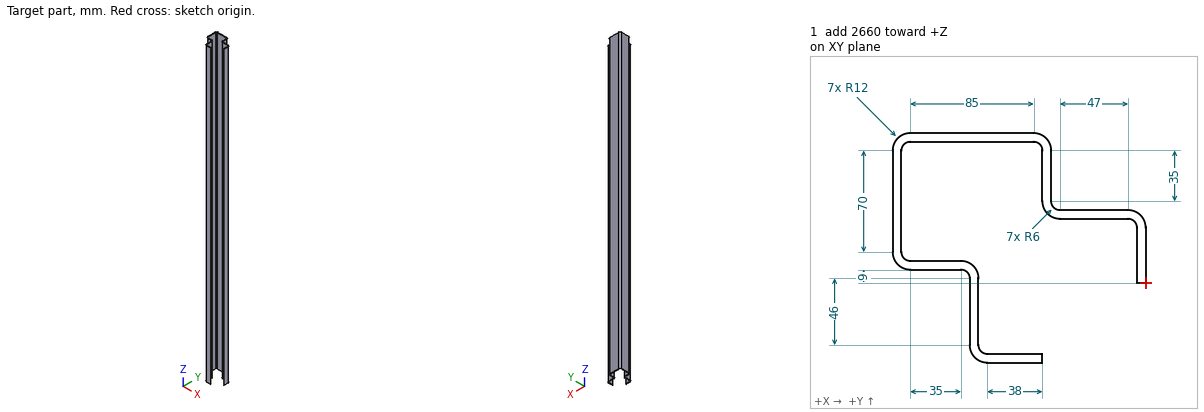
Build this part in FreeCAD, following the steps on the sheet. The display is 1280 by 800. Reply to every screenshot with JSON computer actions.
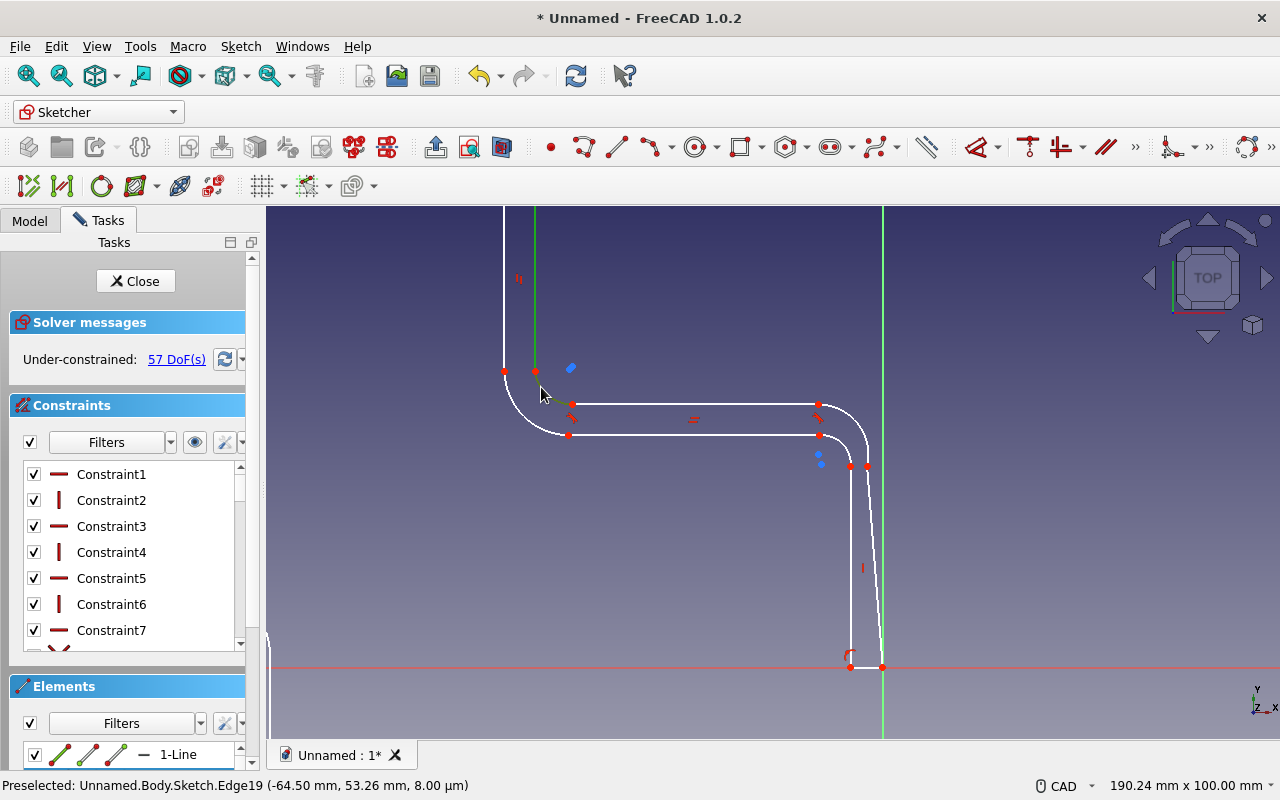
{"action": "key", "text": "t"}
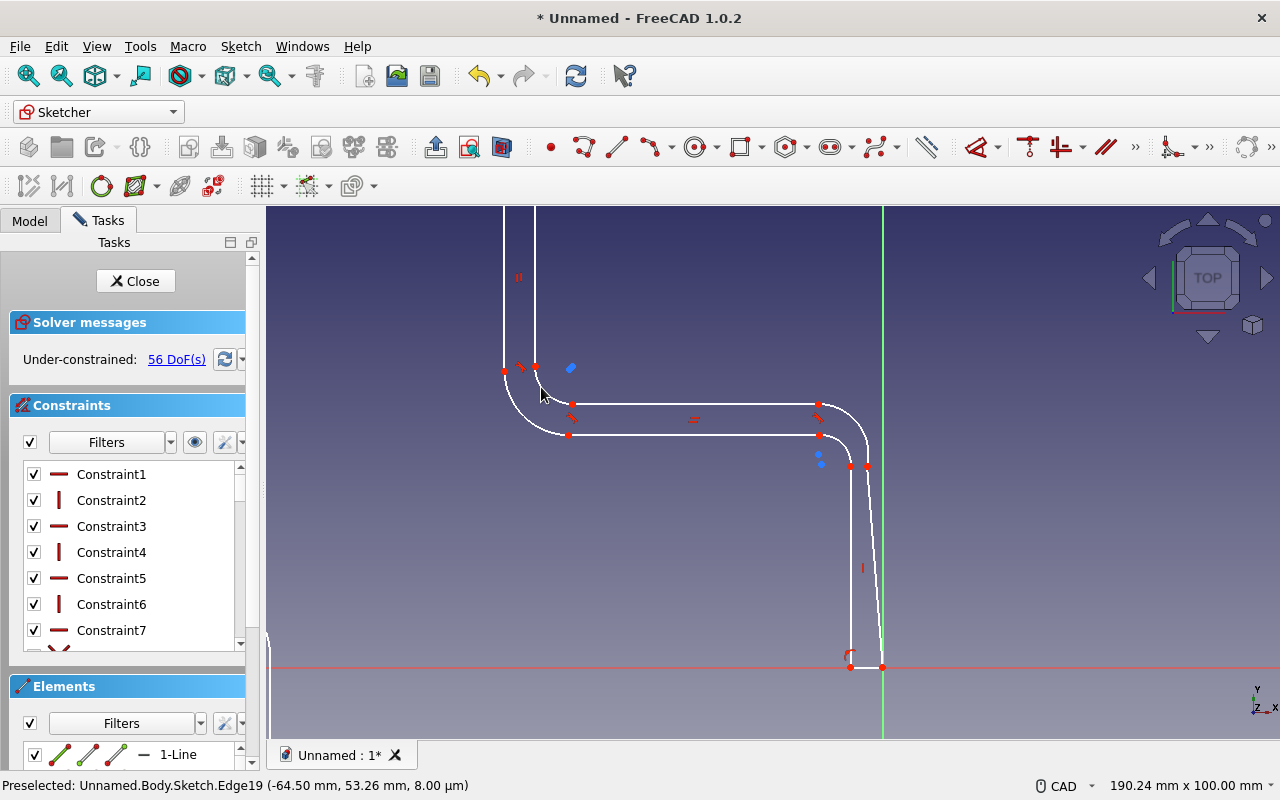
{"action": "left_click", "coordinate": [535, 313]}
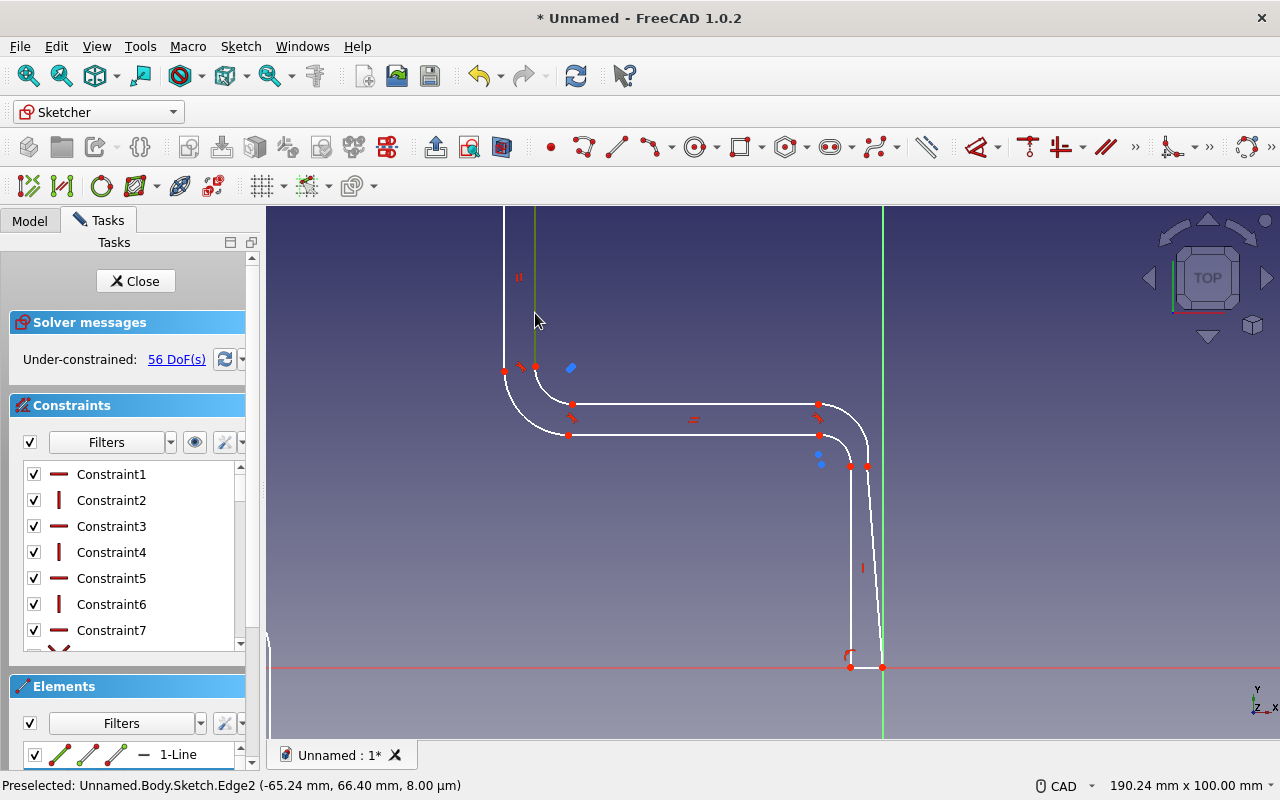
{"action": "scroll", "coordinate": [871, 433], "scroll_direction": "down", "scroll_amount": 5}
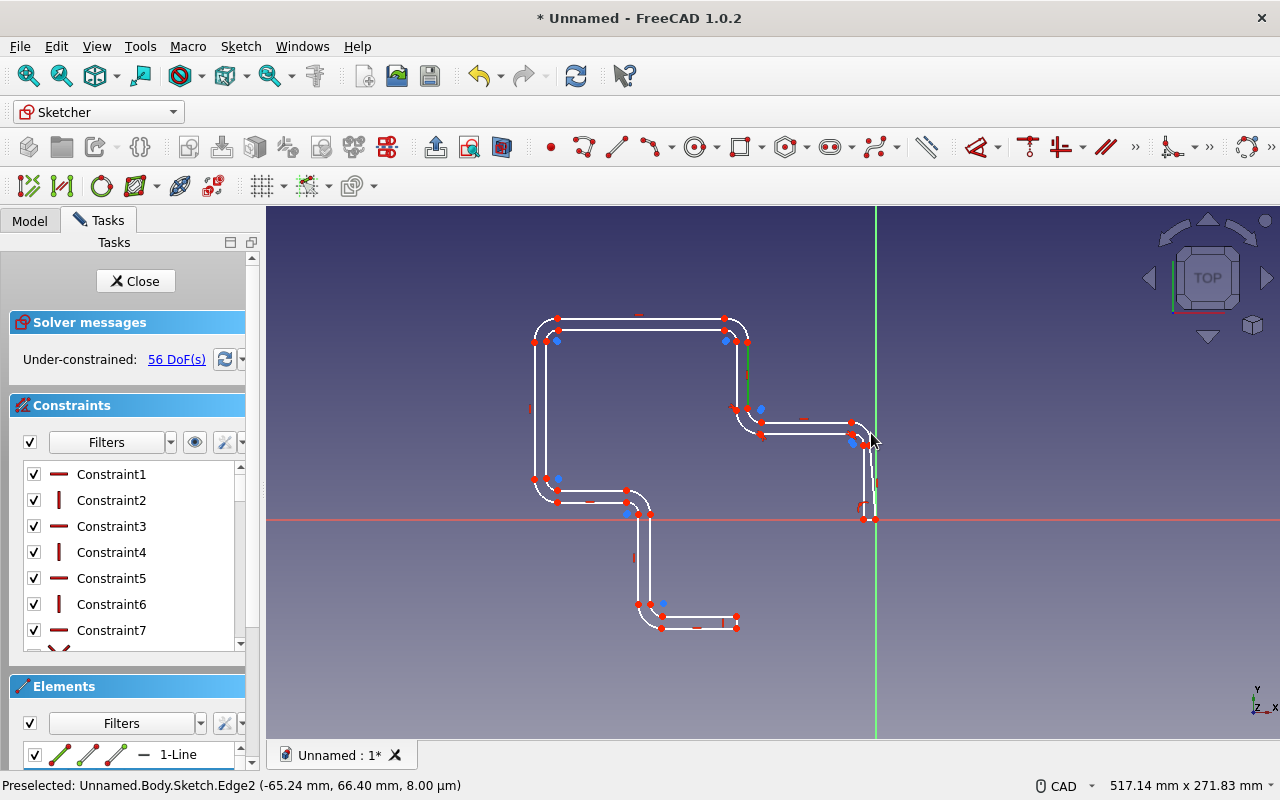
{"action": "scroll", "coordinate": [746, 332], "scroll_direction": "up", "scroll_amount": 2}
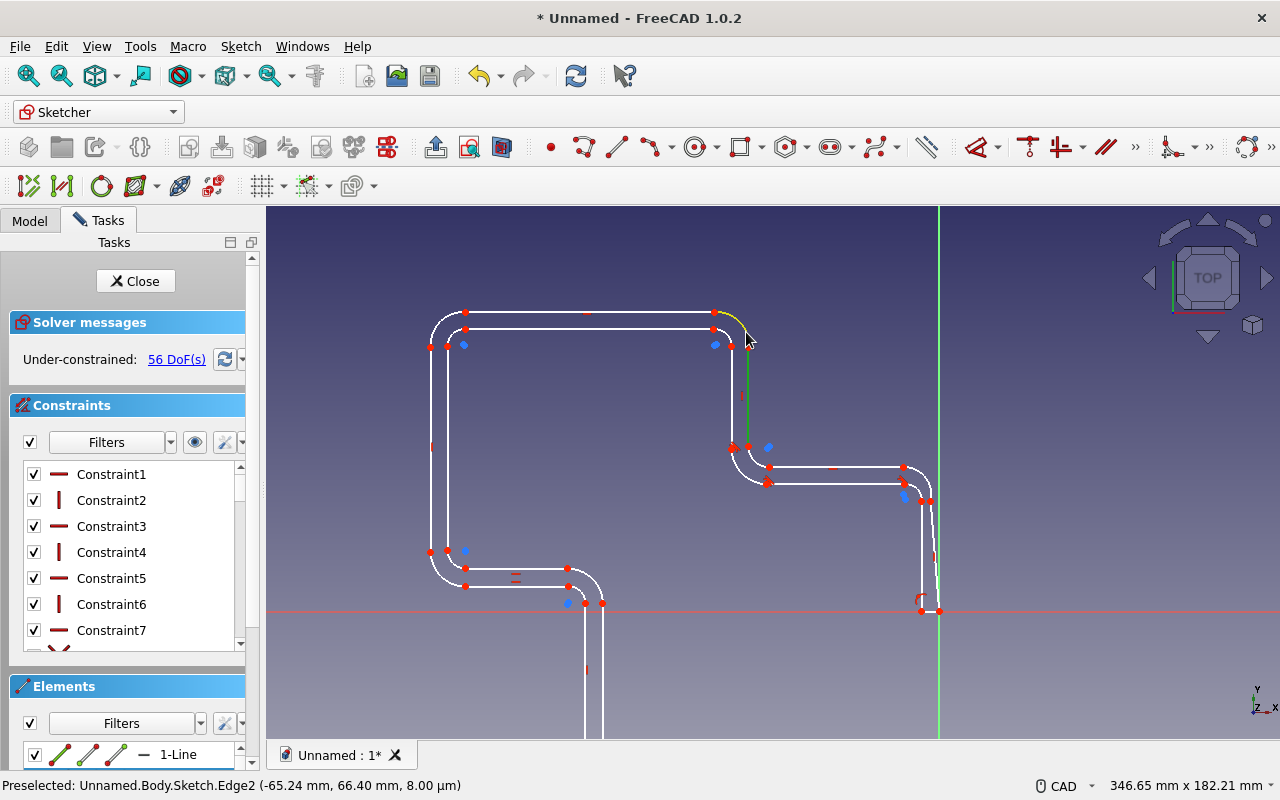
{"action": "left_click", "coordinate": [746, 331]}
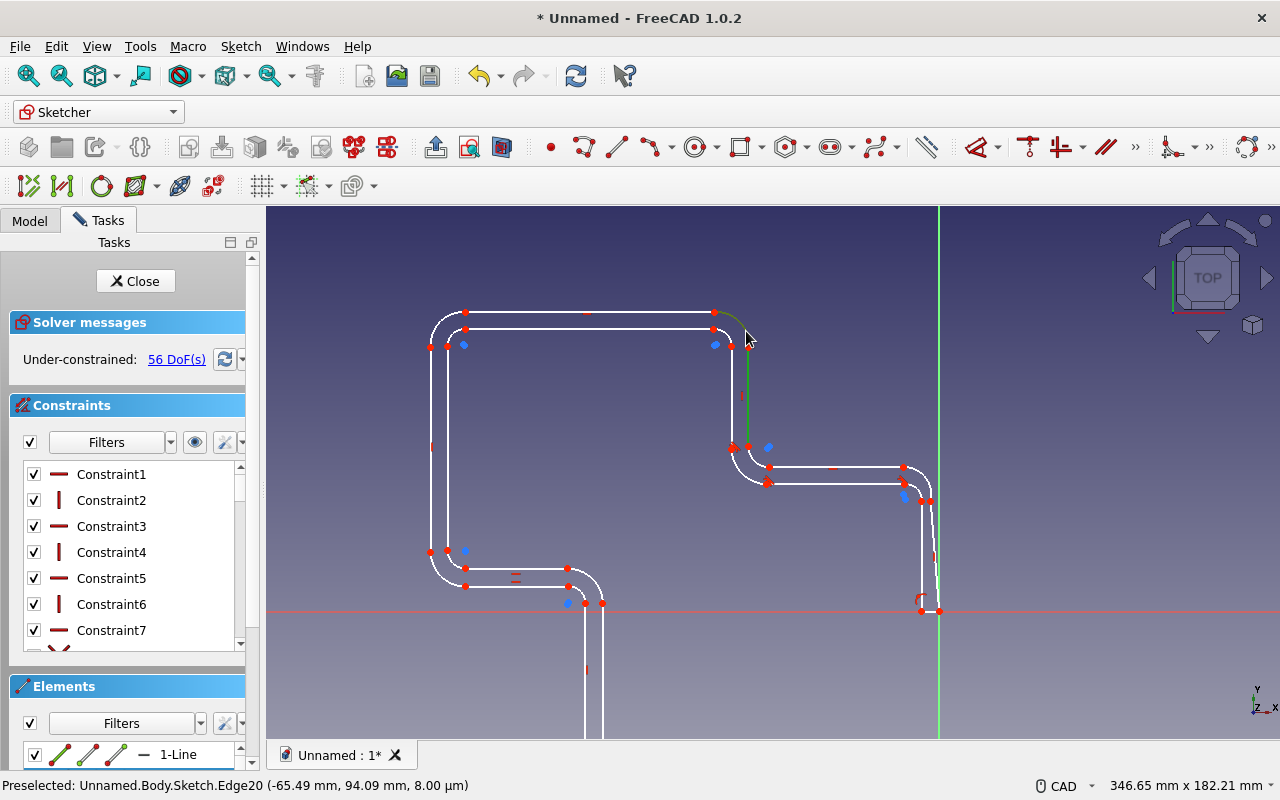
{"action": "key", "text": "t"}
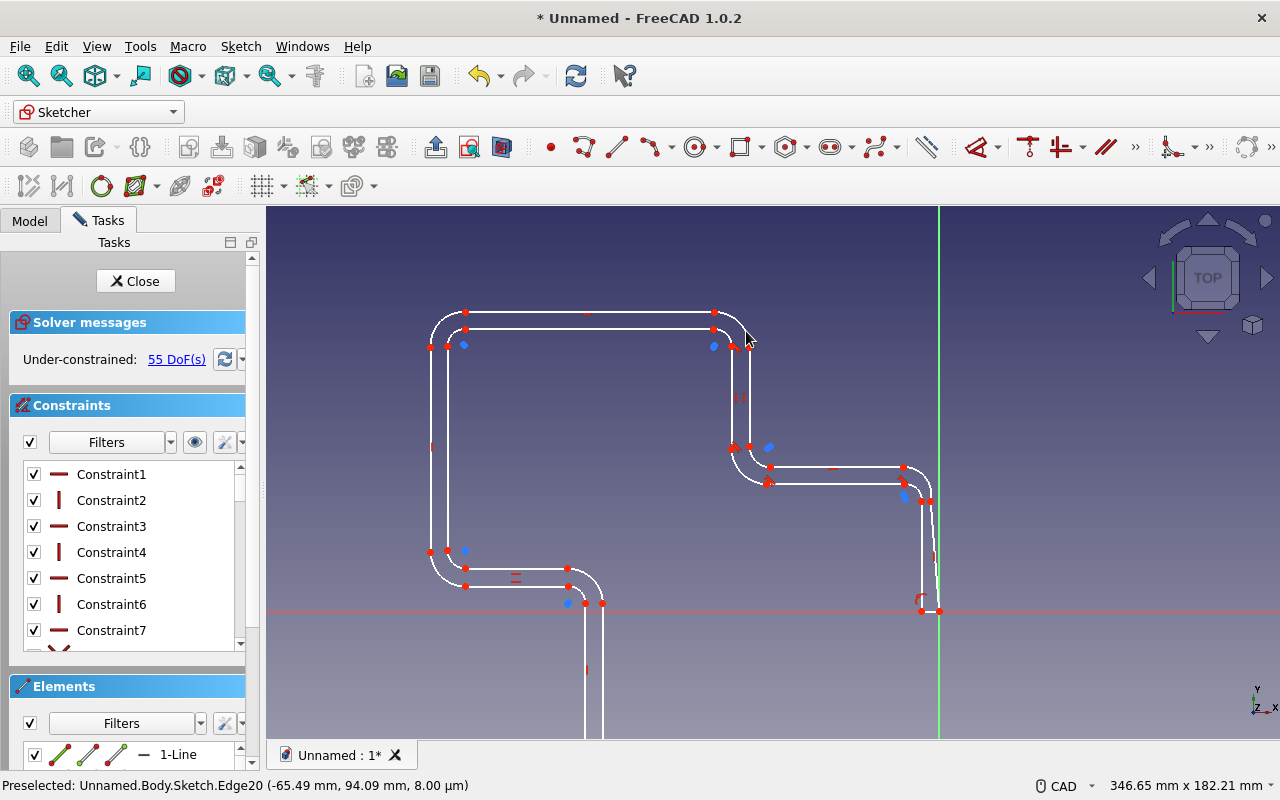
{"action": "left_click", "coordinate": [640, 312]}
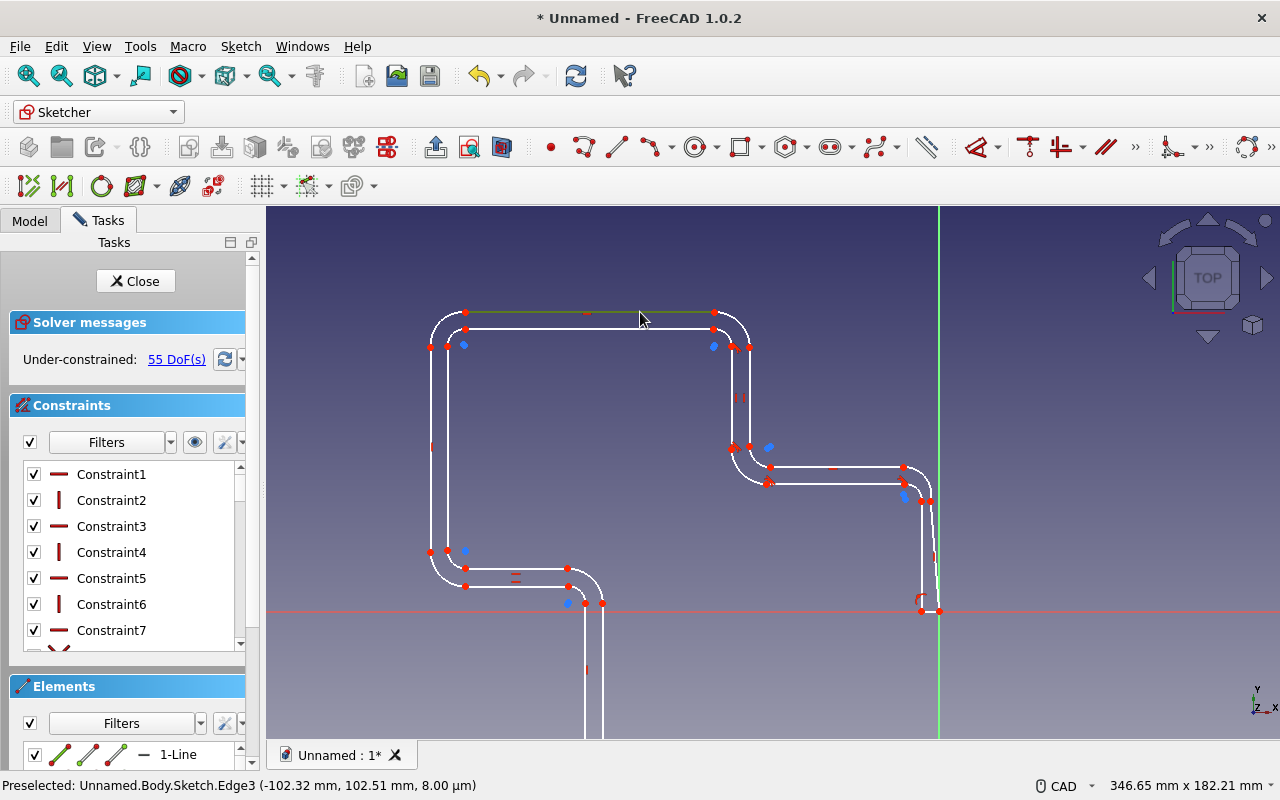
{"action": "left_click", "coordinate": [746, 332]}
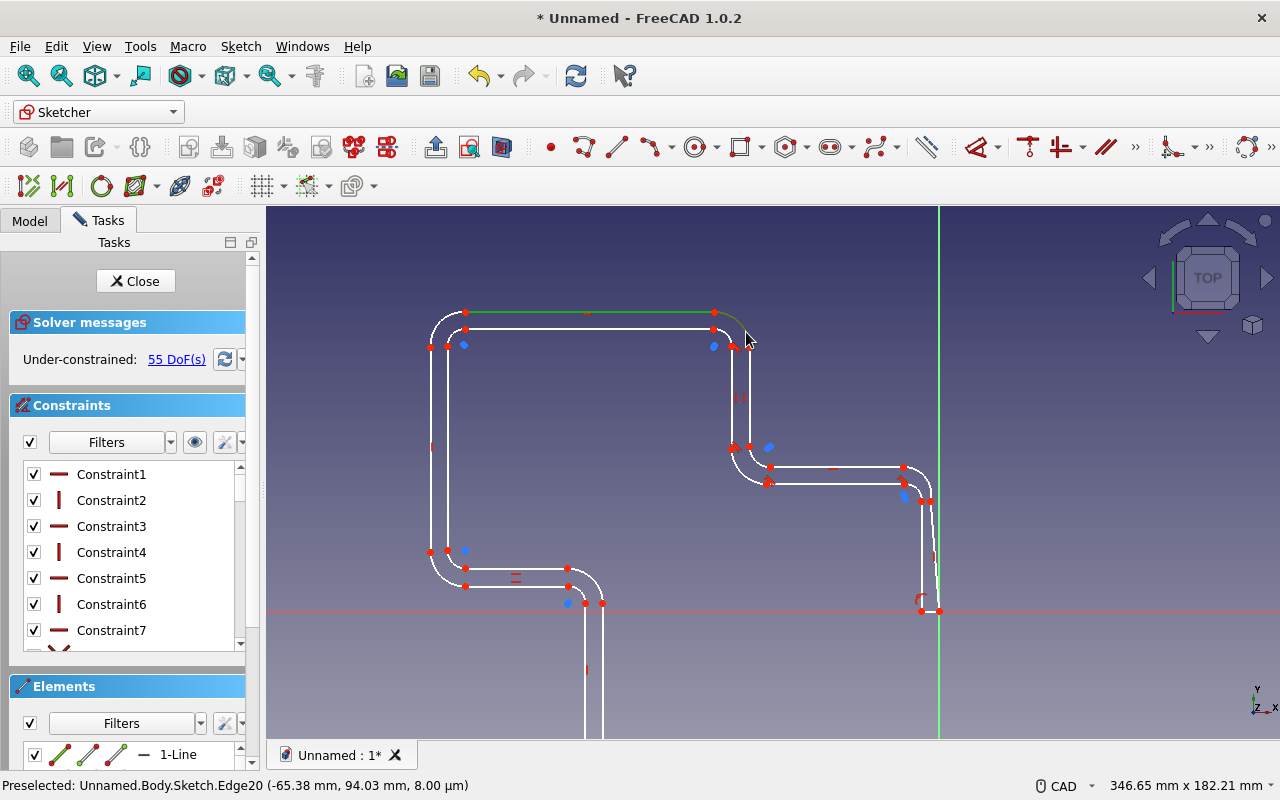
{"action": "key", "text": "t"}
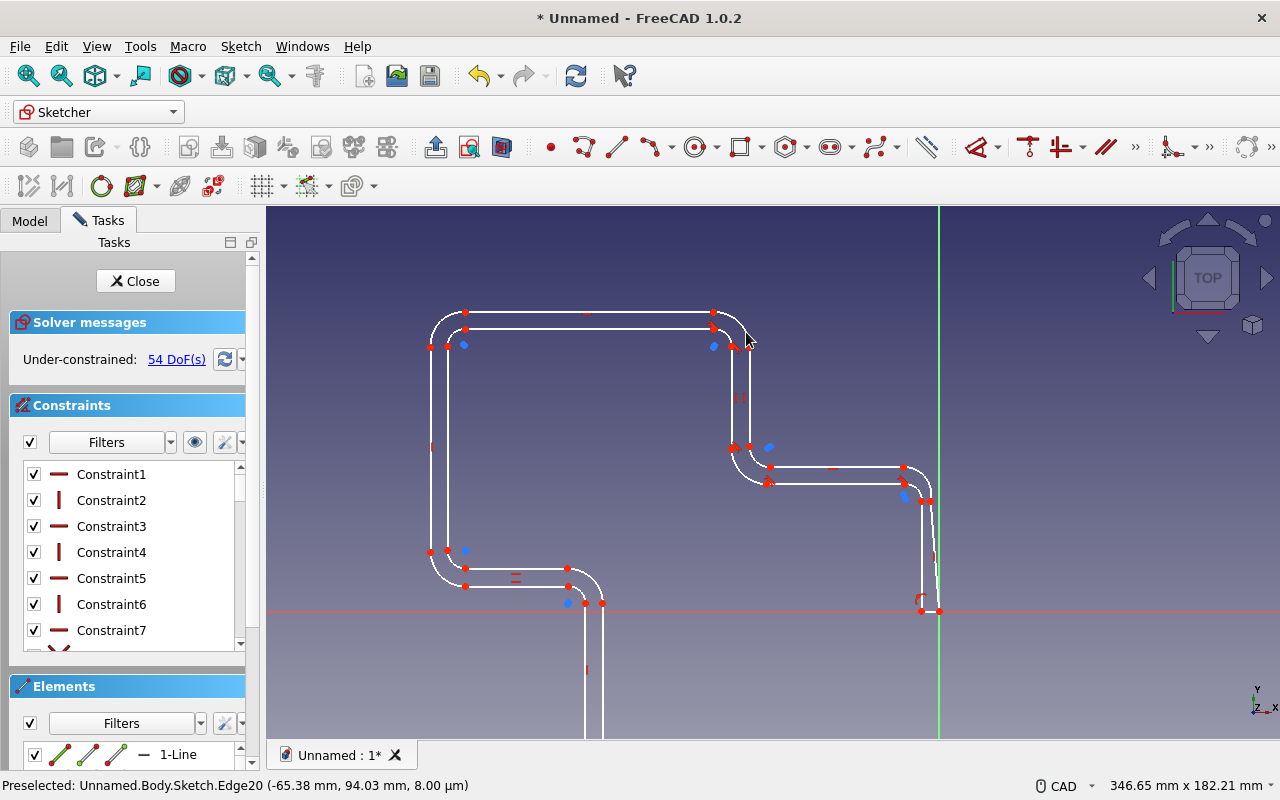
{"action": "left_click", "coordinate": [639, 312]}